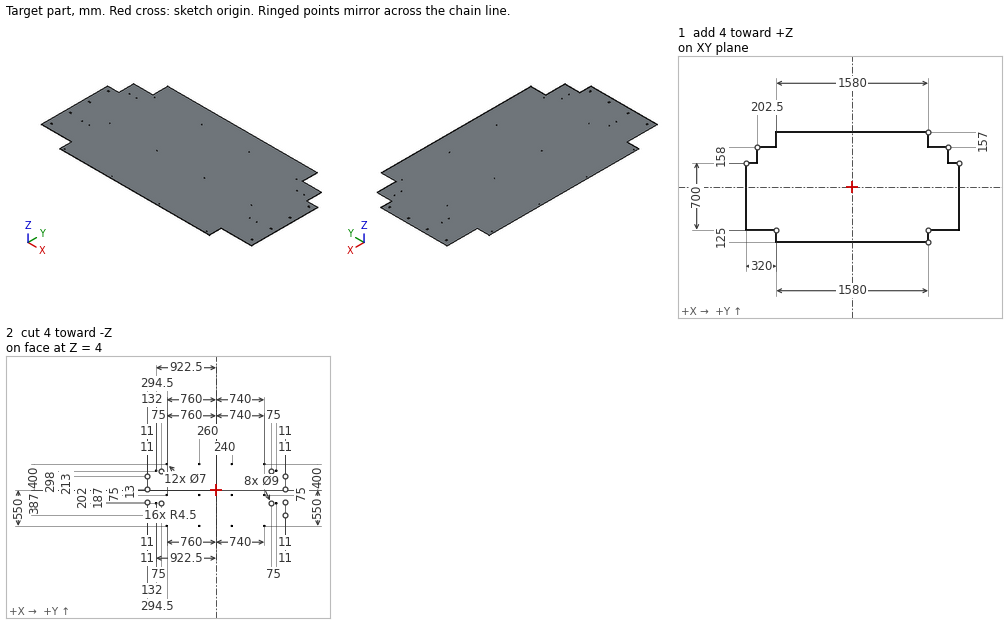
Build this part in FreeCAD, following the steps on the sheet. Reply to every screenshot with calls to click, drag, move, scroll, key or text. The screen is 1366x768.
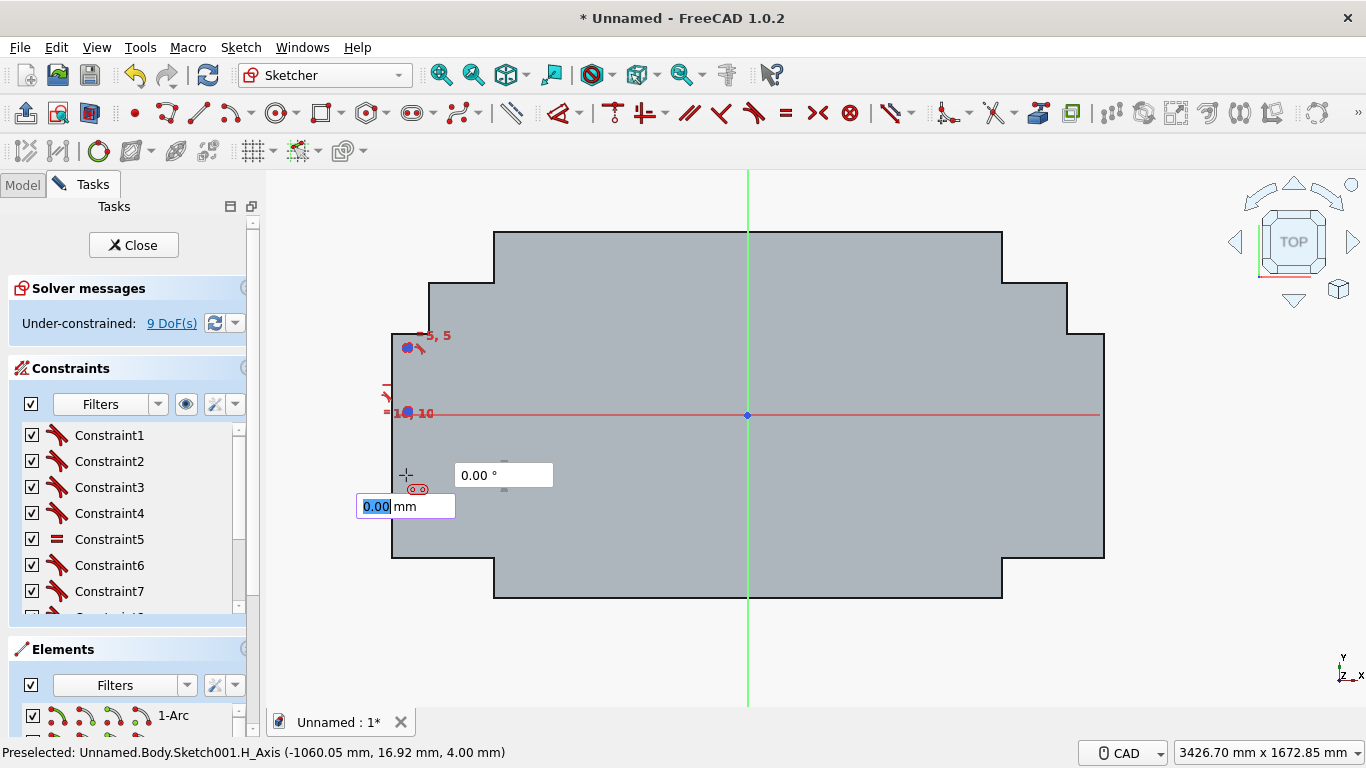
scroll(409, 475, up, 8)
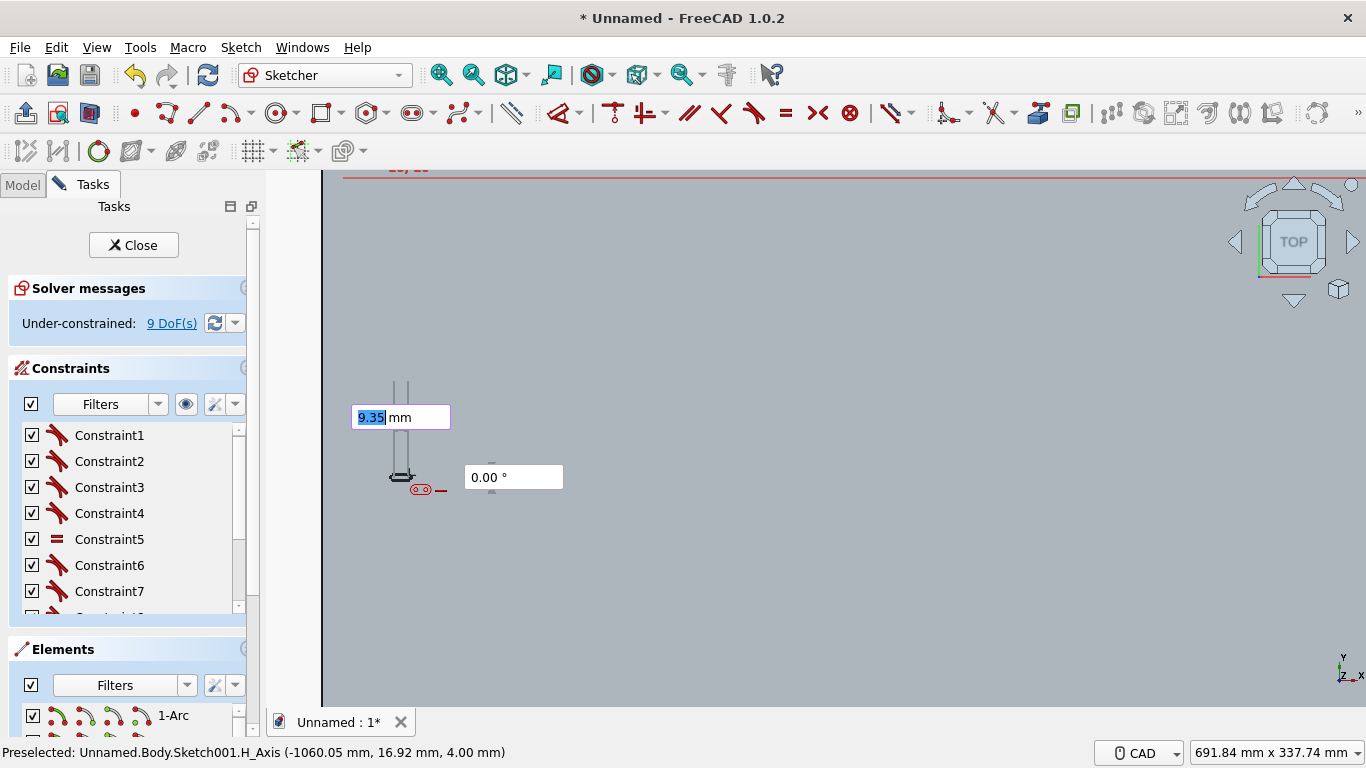
click(411, 473)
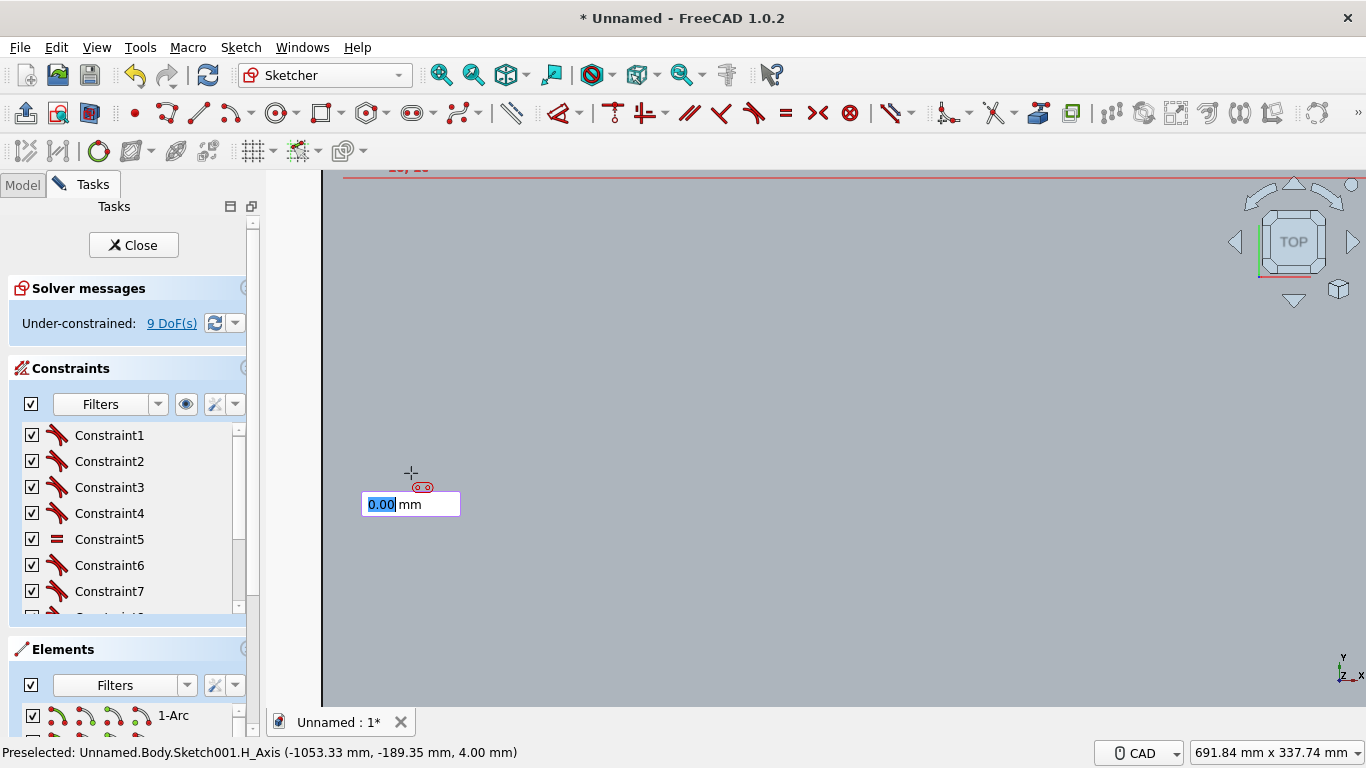
scroll(402, 468, up, 4)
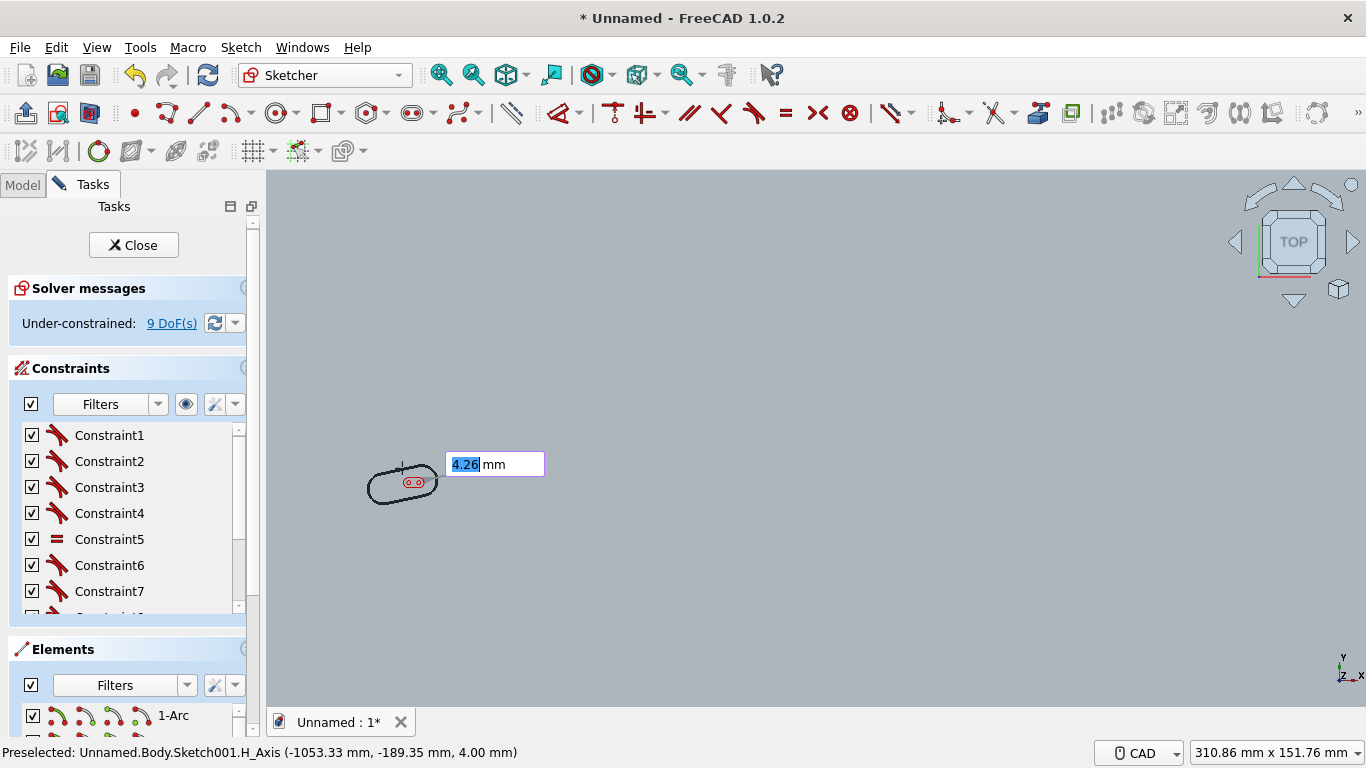
click(402, 467)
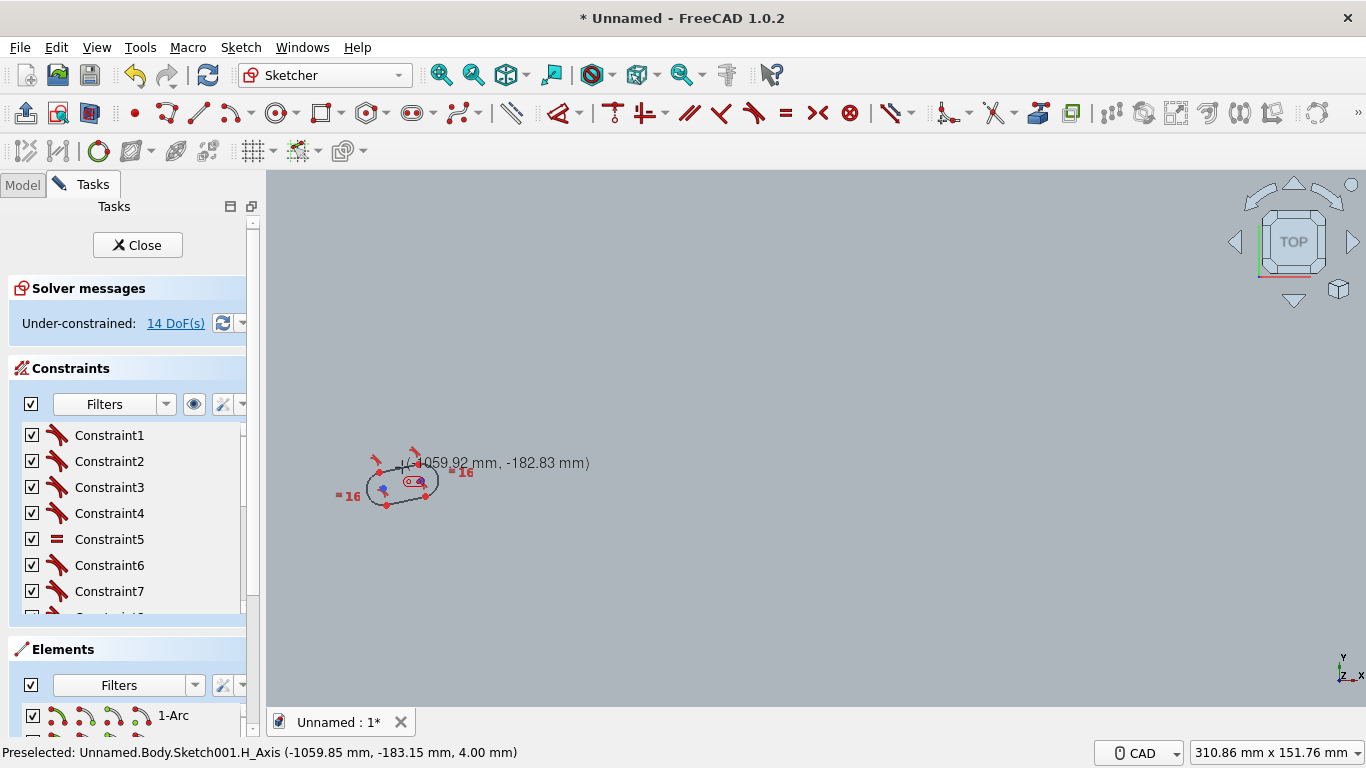
scroll(408, 474, down, 12)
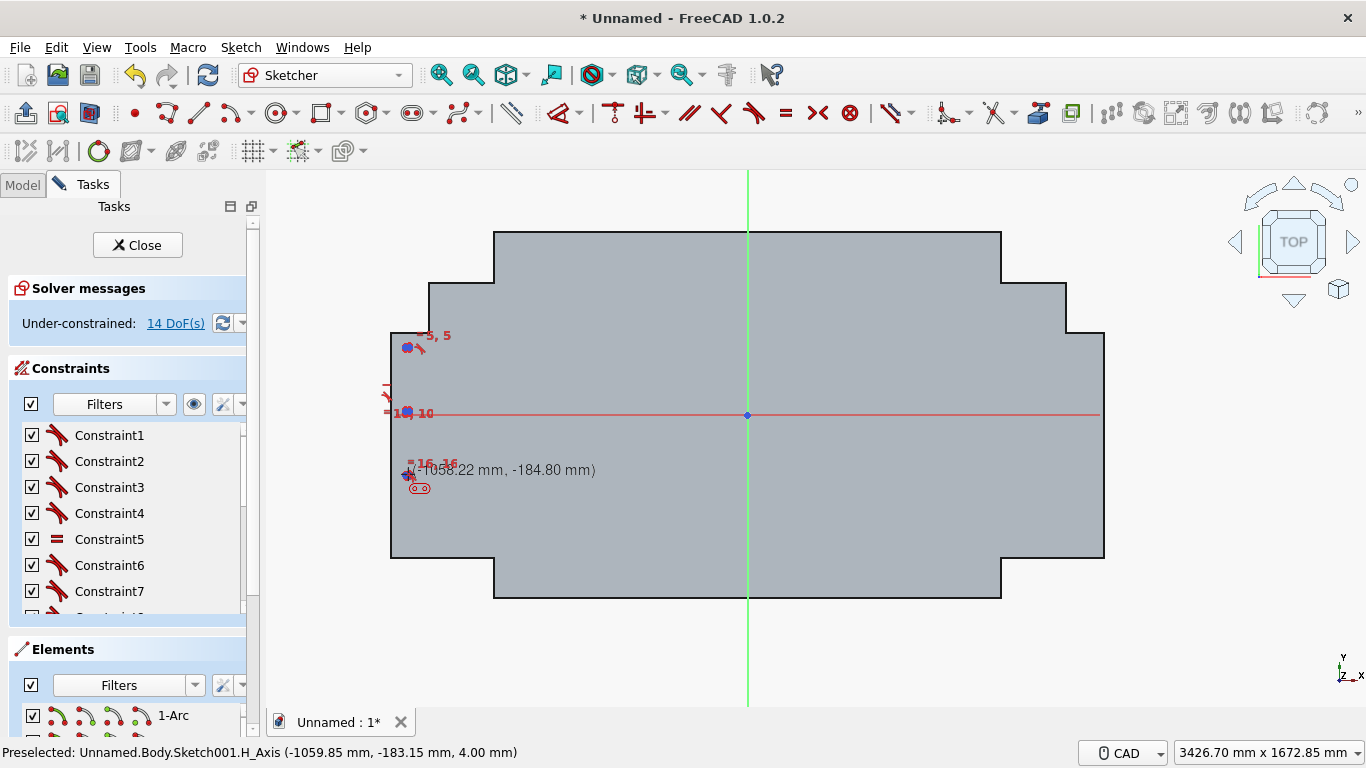
scroll(406, 540, up, 14)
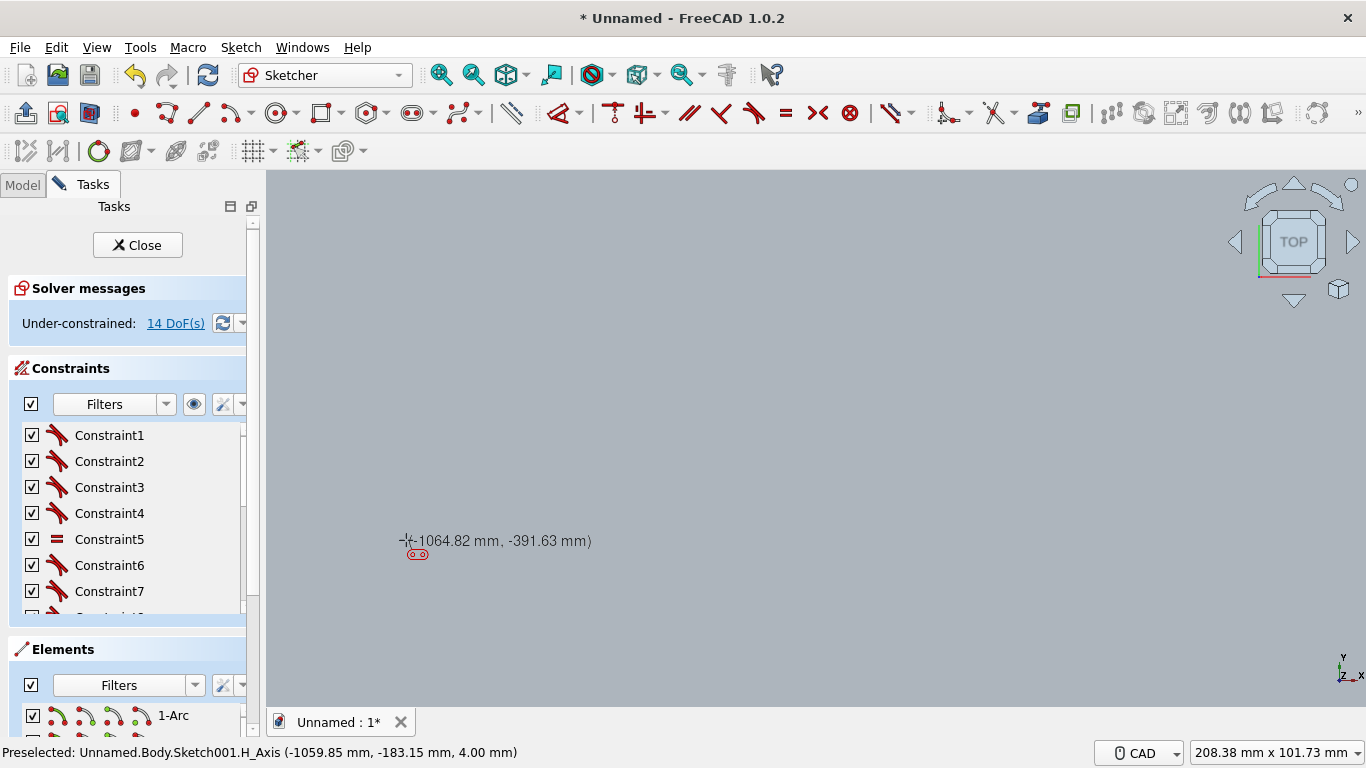
scroll(406, 540, down, 14)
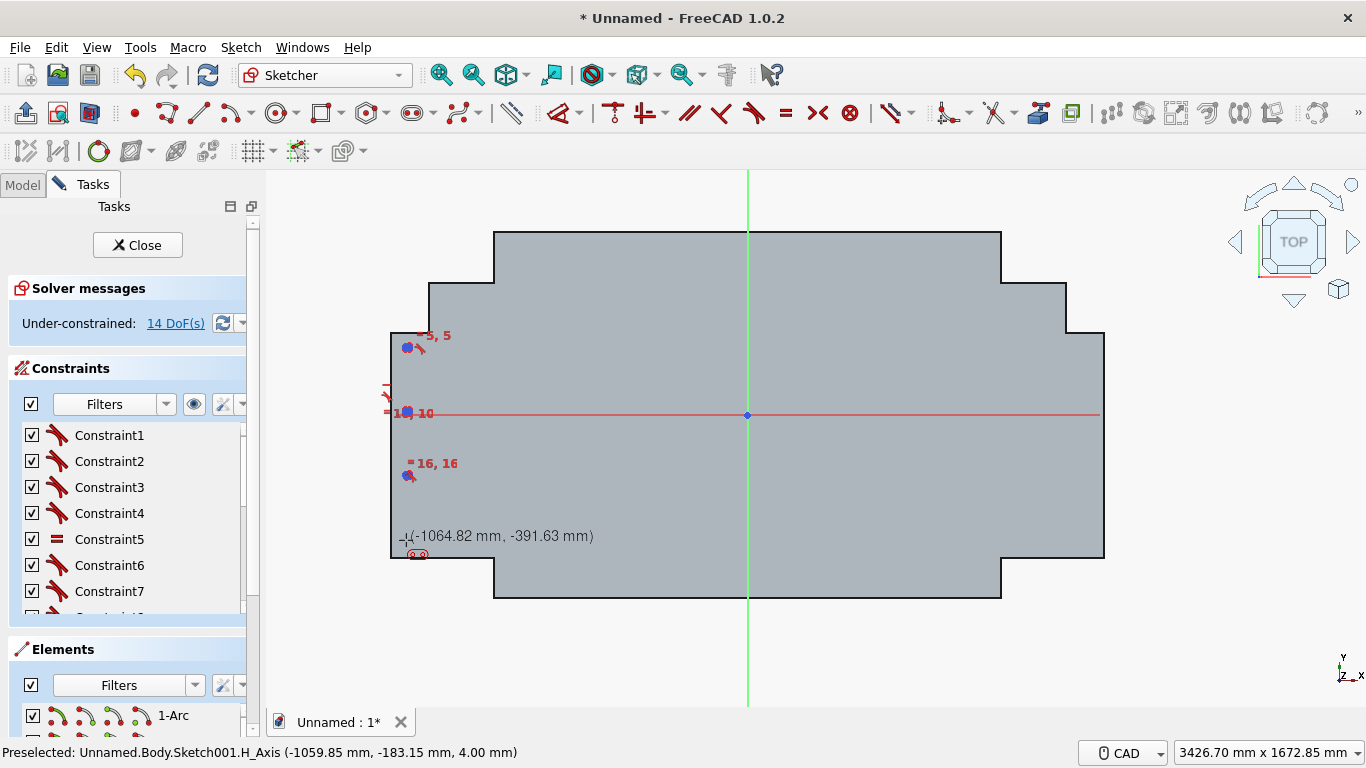
click(406, 540)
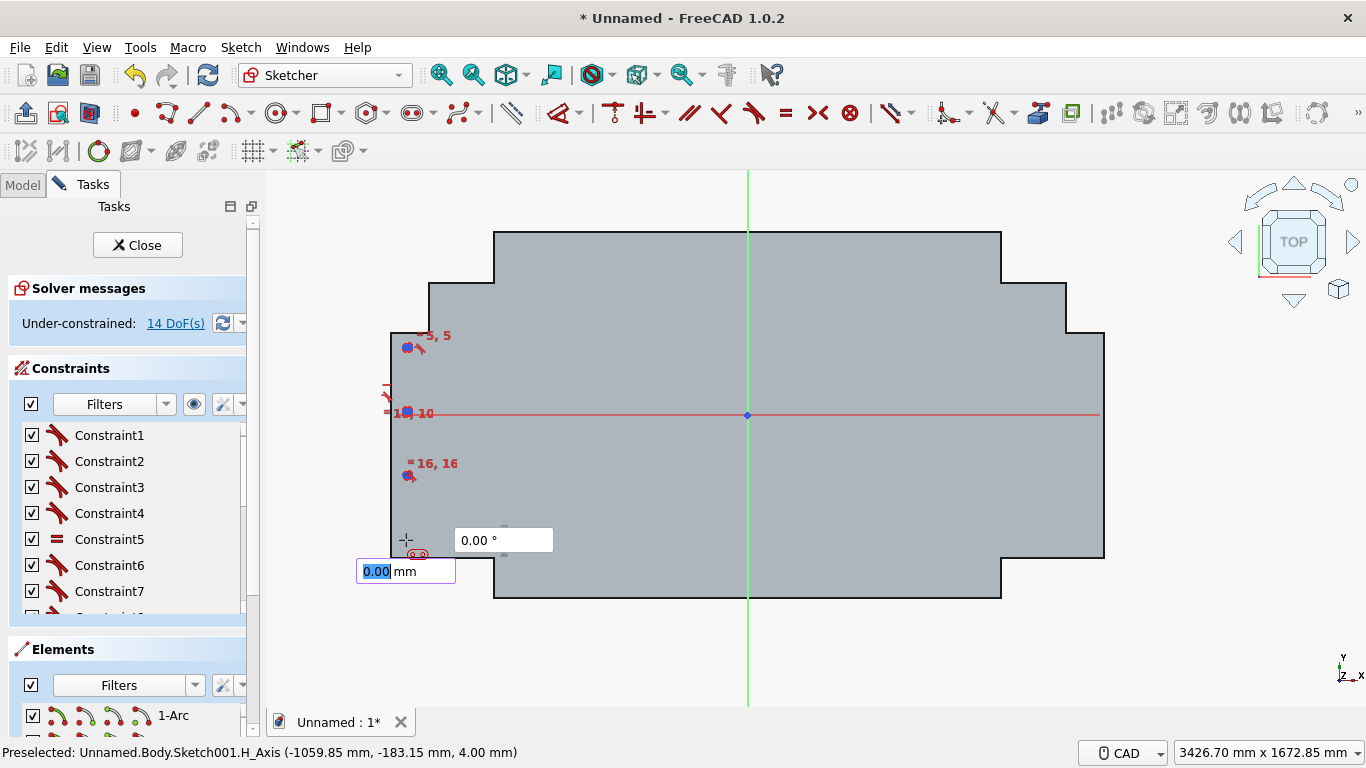
scroll(409, 540, up, 8)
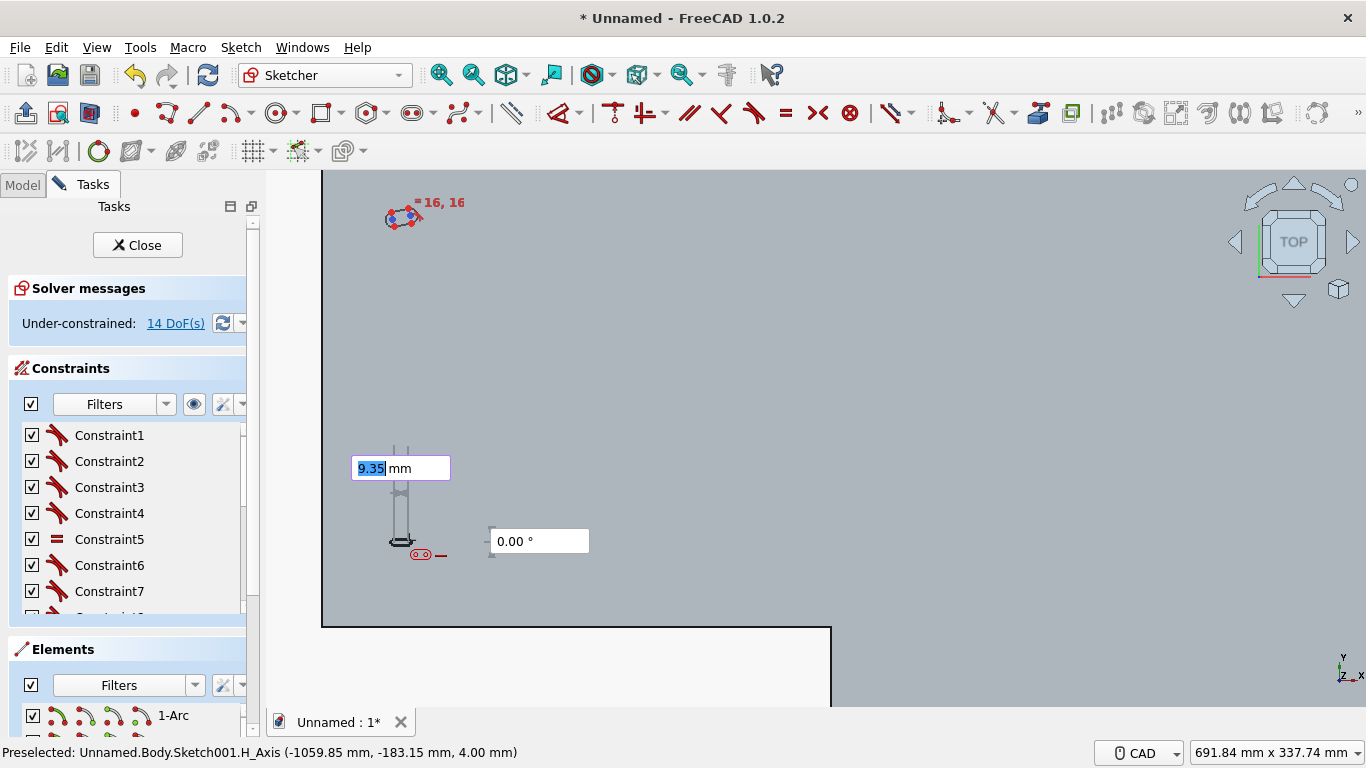
click(410, 537)